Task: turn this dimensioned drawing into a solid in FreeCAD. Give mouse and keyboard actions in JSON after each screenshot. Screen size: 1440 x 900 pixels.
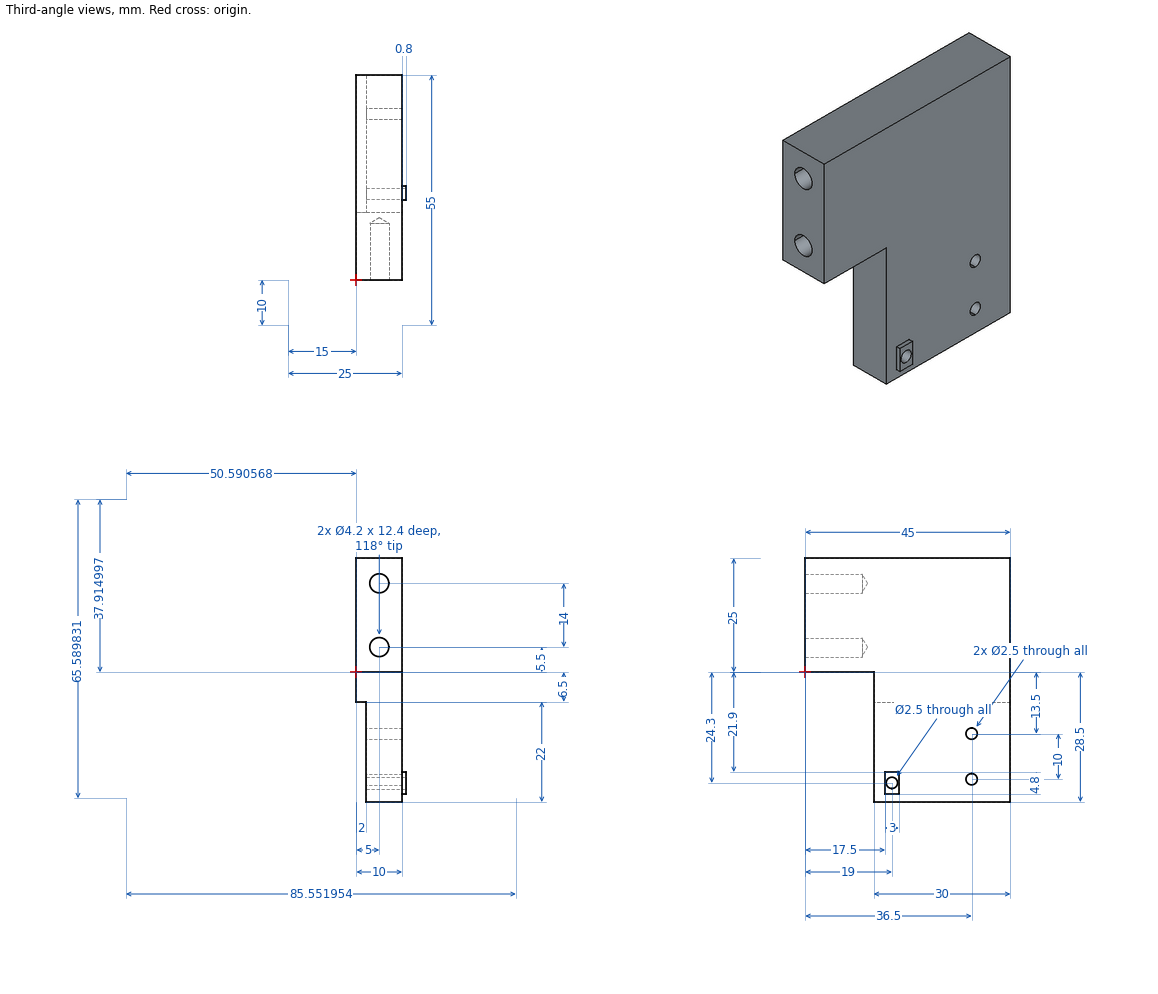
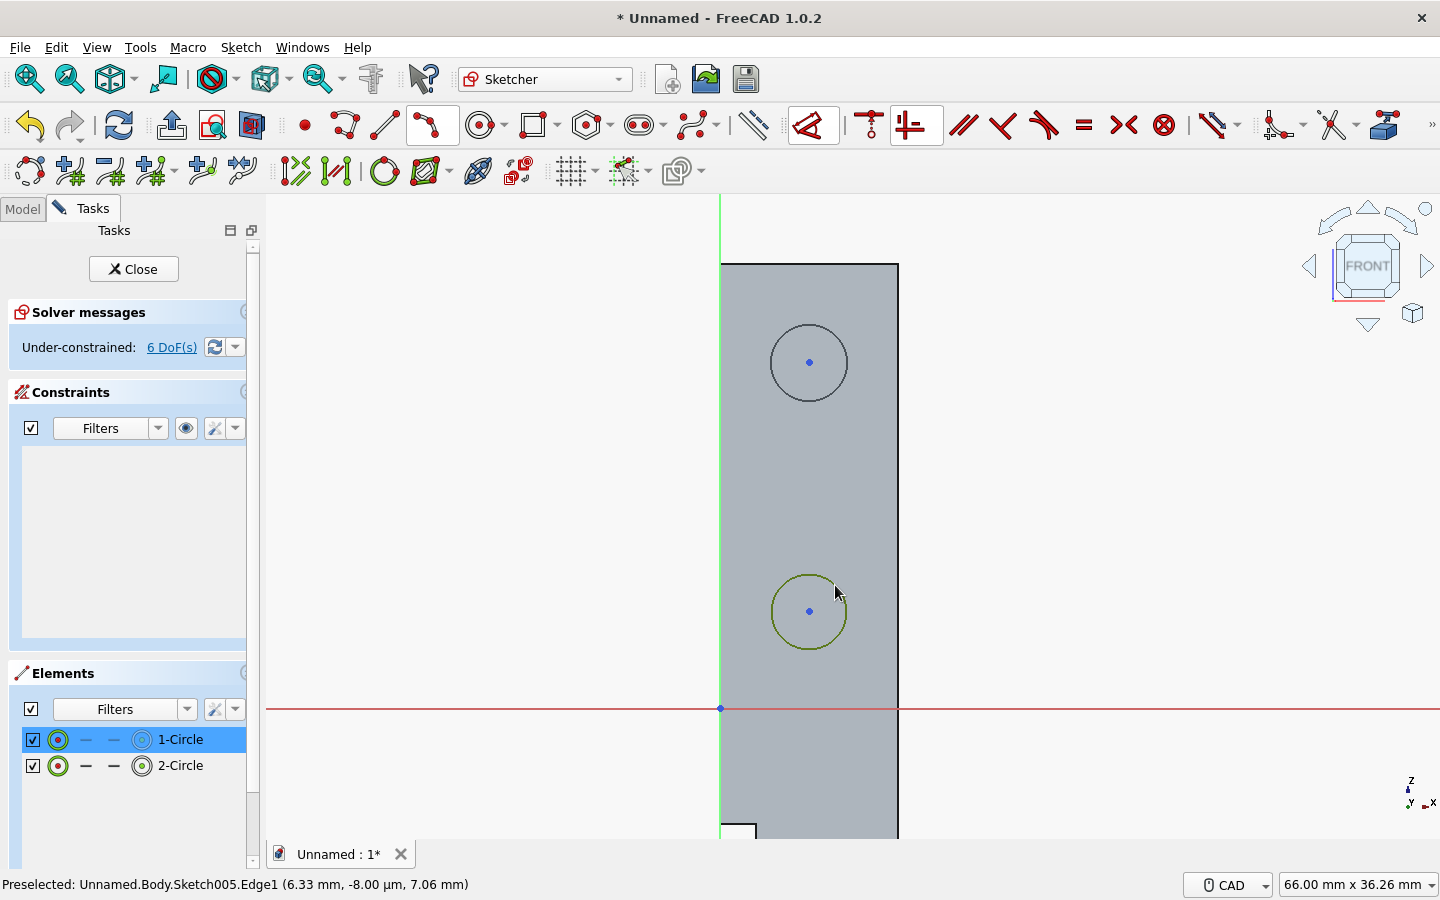
{"action": "left_click", "coordinate": [836, 336]}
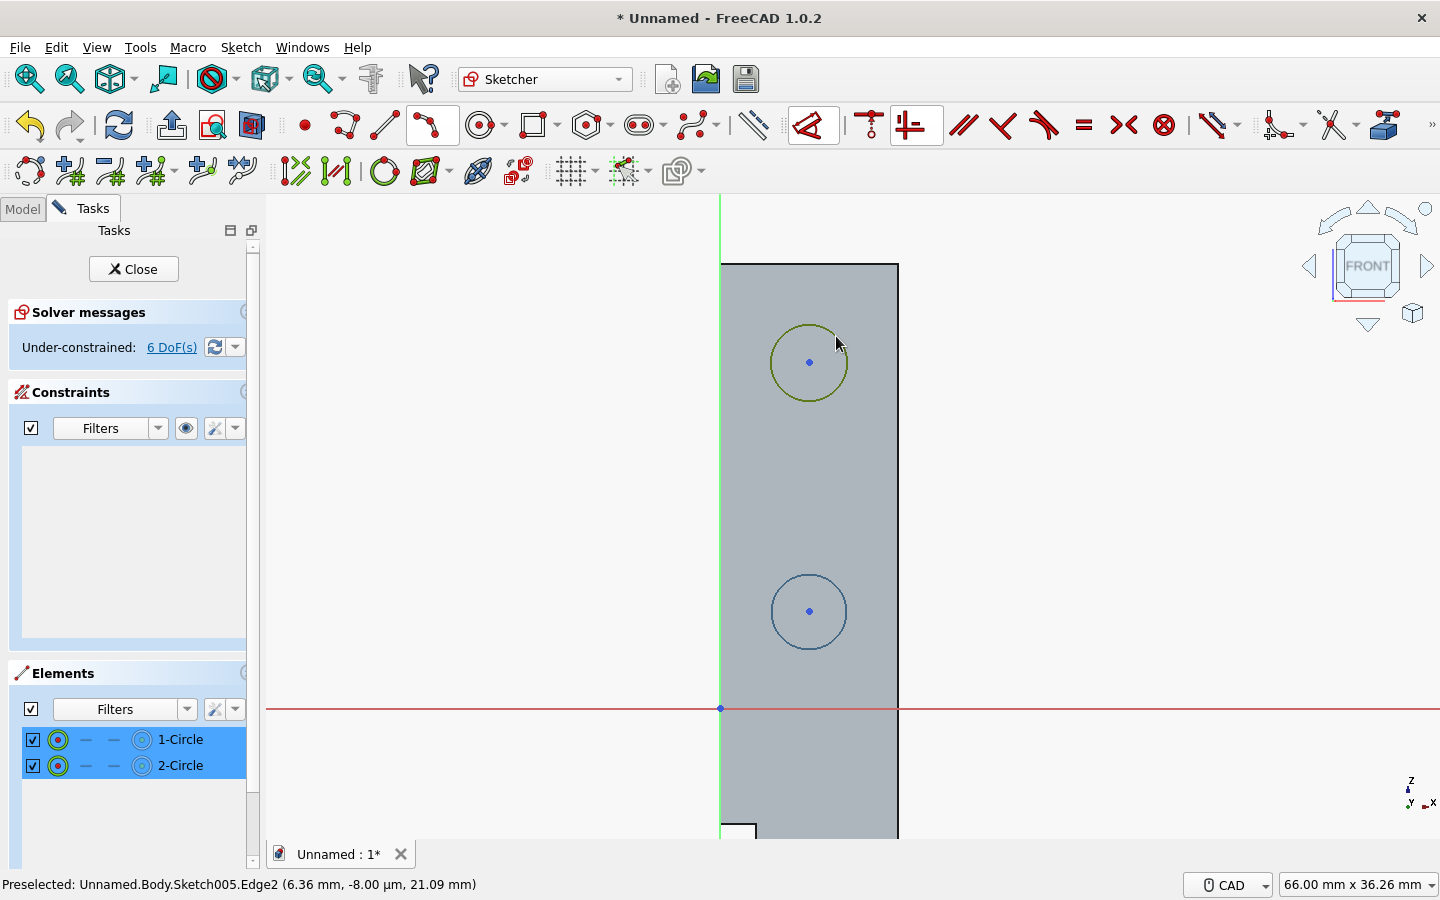
{"action": "left_click", "coordinate": [1084, 126]}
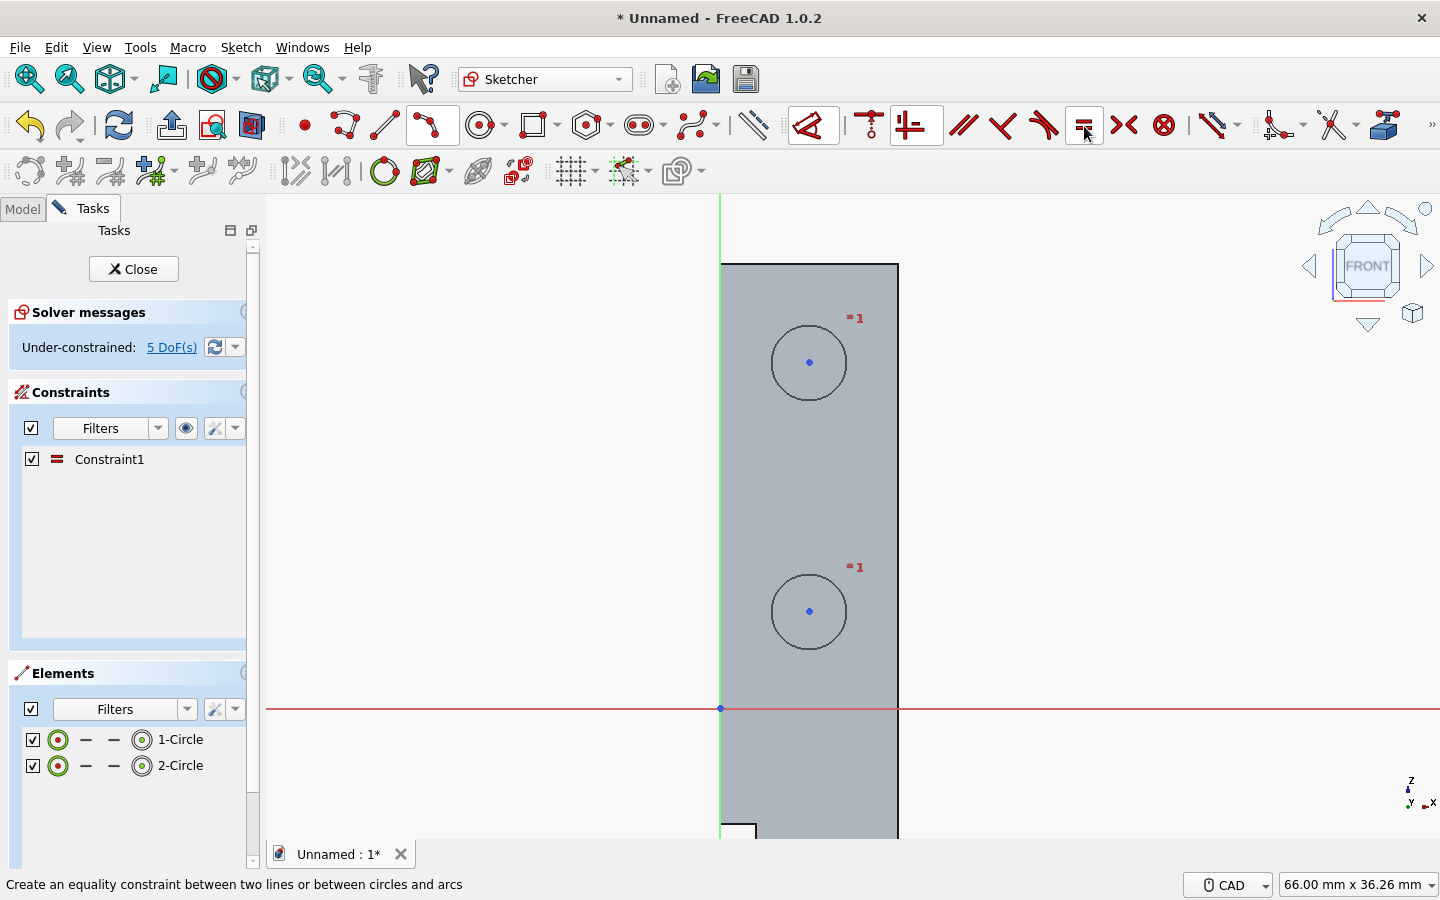
{"action": "left_click", "coordinate": [809, 612]}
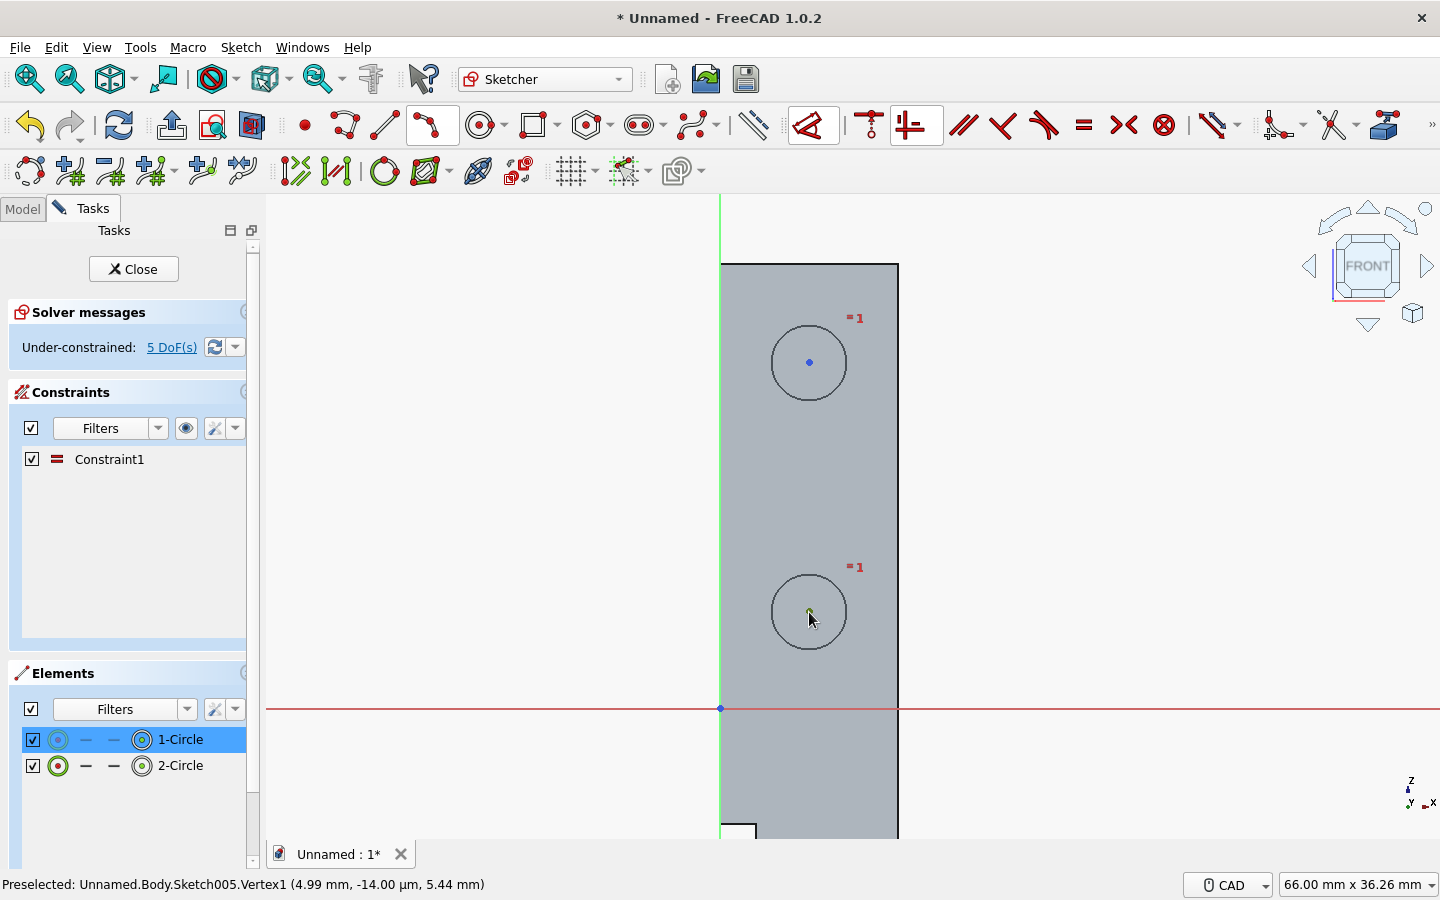
{"action": "left_click", "coordinate": [809, 363]}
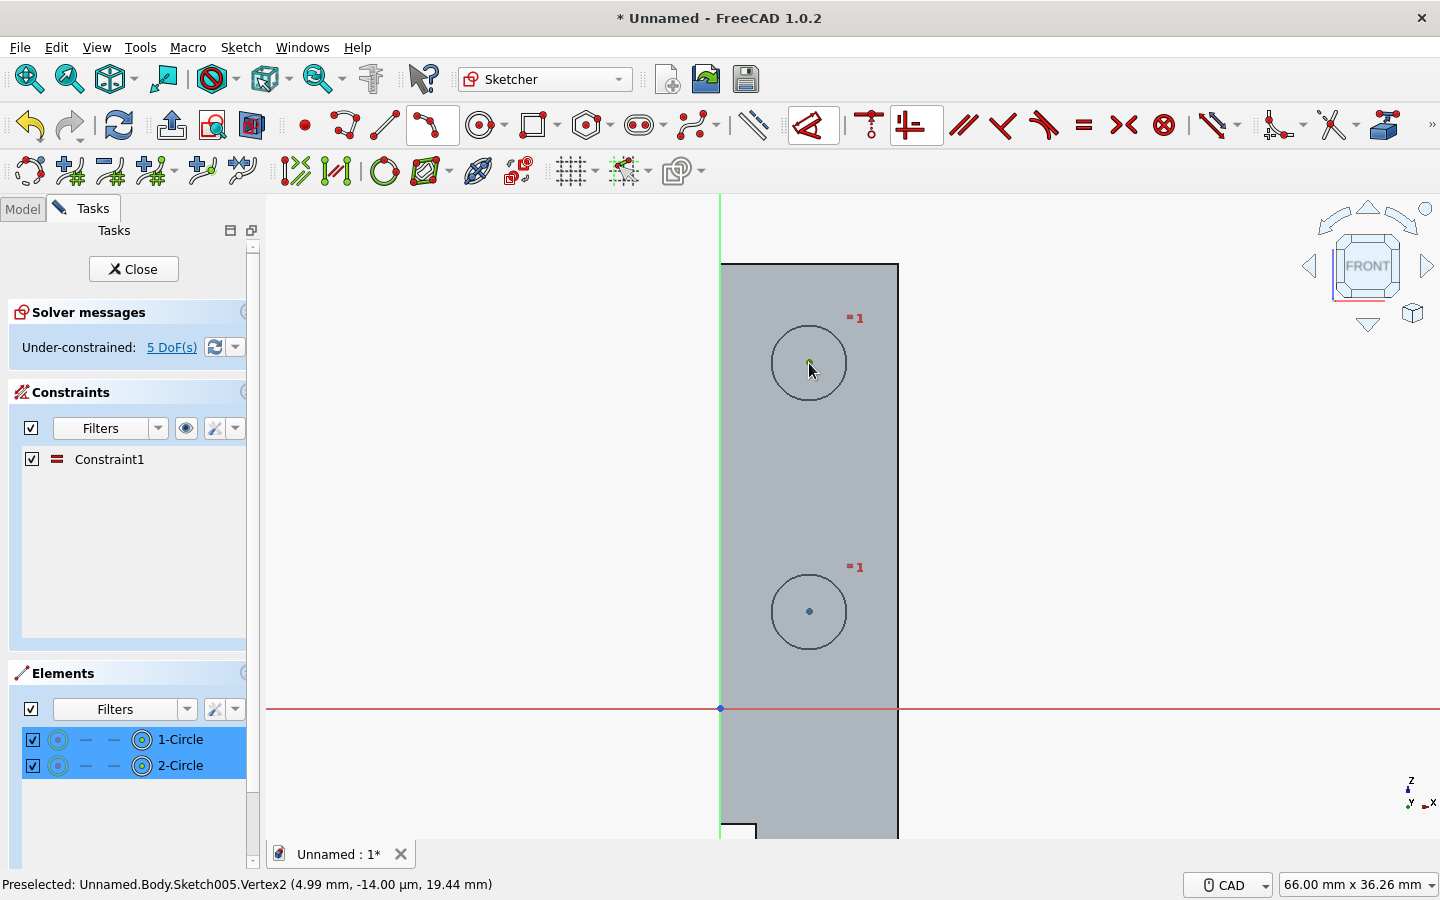
{"action": "key", "text": "v"}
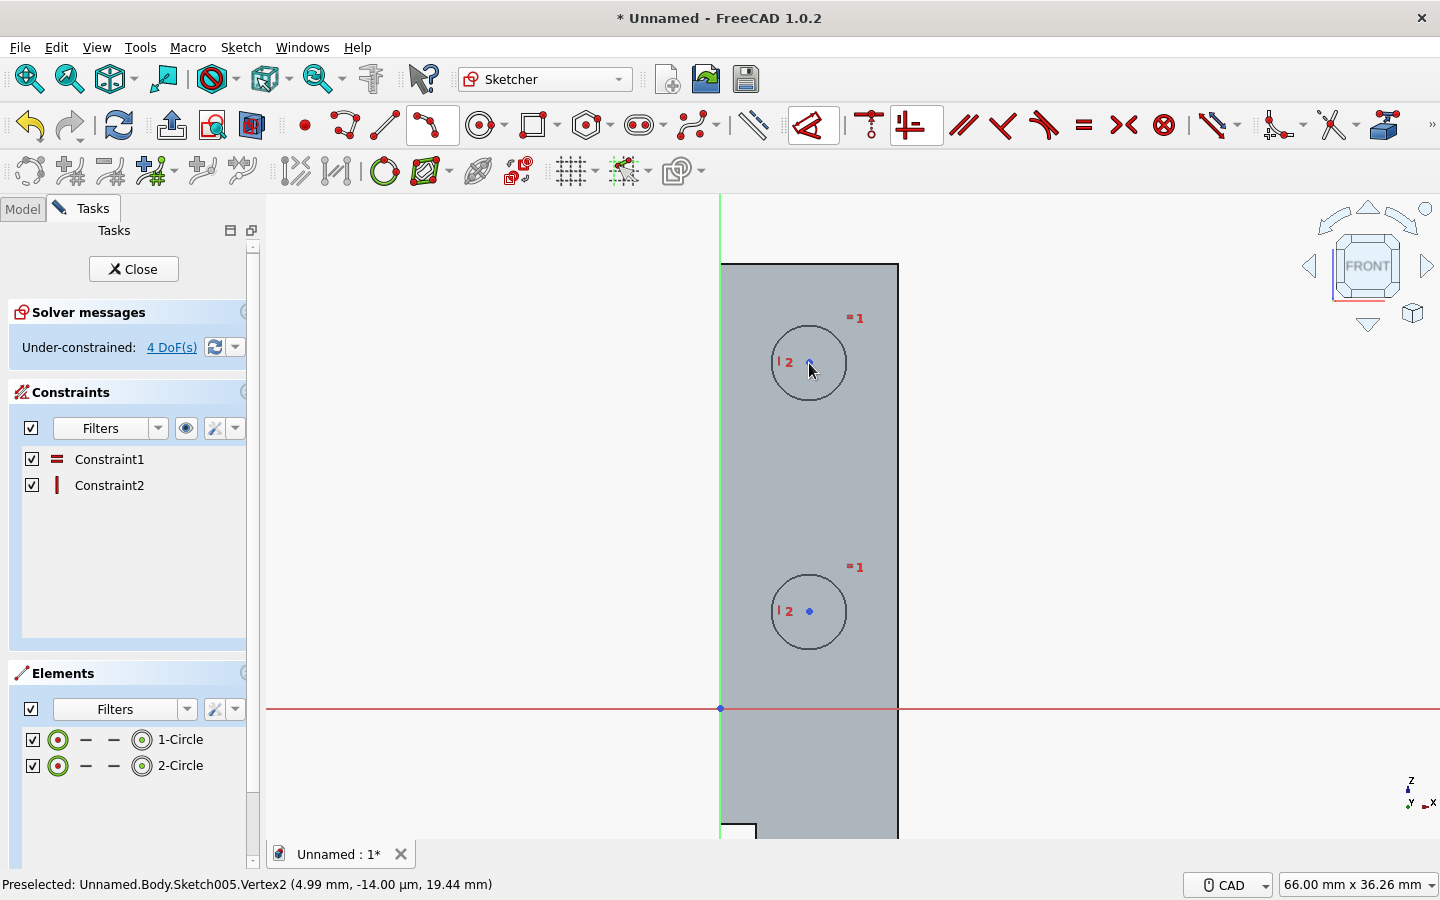
{"action": "left_click", "coordinate": [835, 585]}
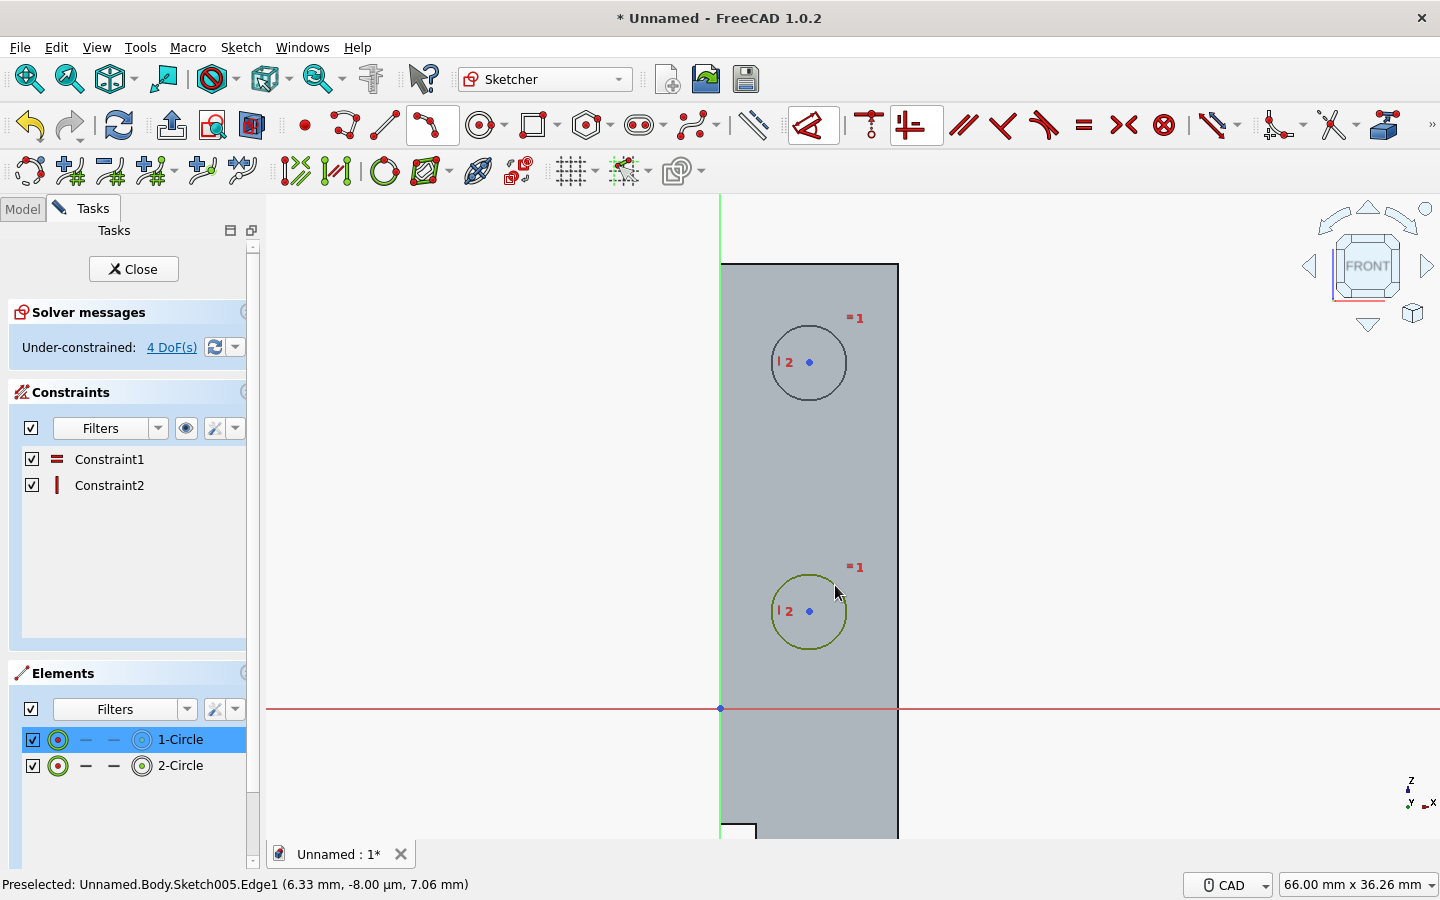
{"action": "left_click", "coordinate": [834, 126]}